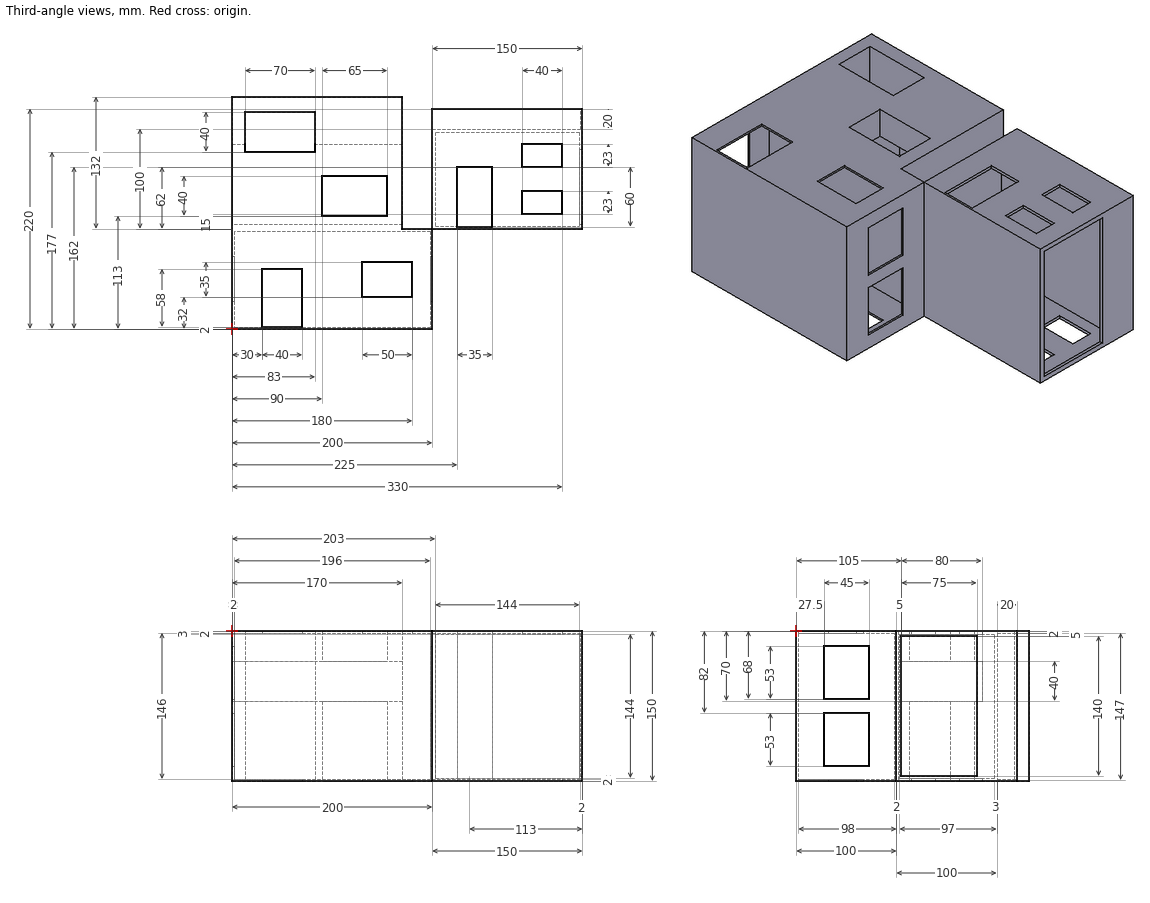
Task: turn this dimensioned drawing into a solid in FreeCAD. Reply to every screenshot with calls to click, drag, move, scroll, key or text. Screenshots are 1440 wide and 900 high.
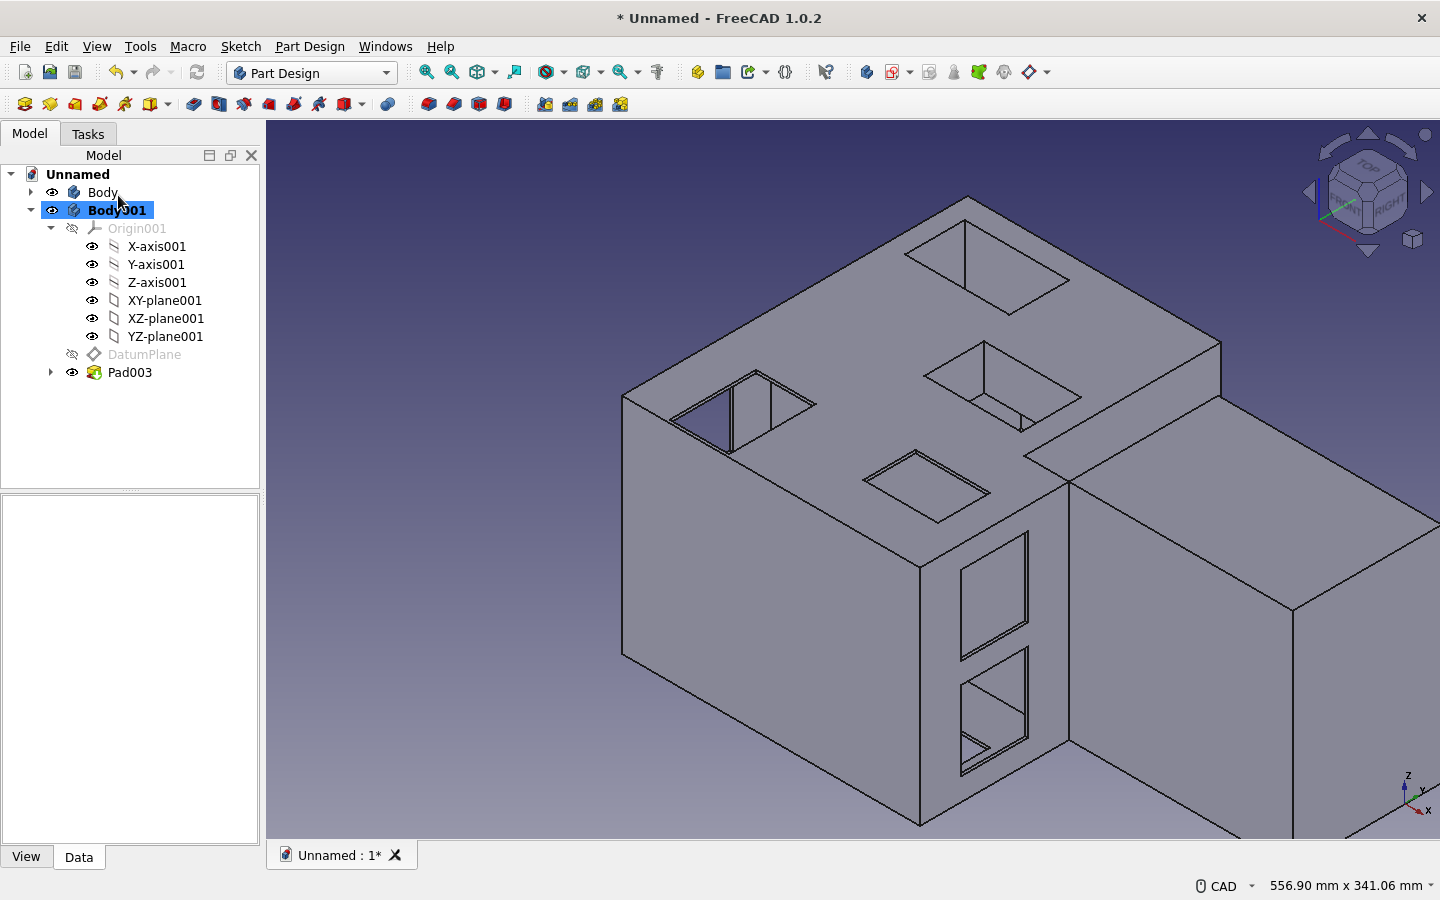
click(427, 72)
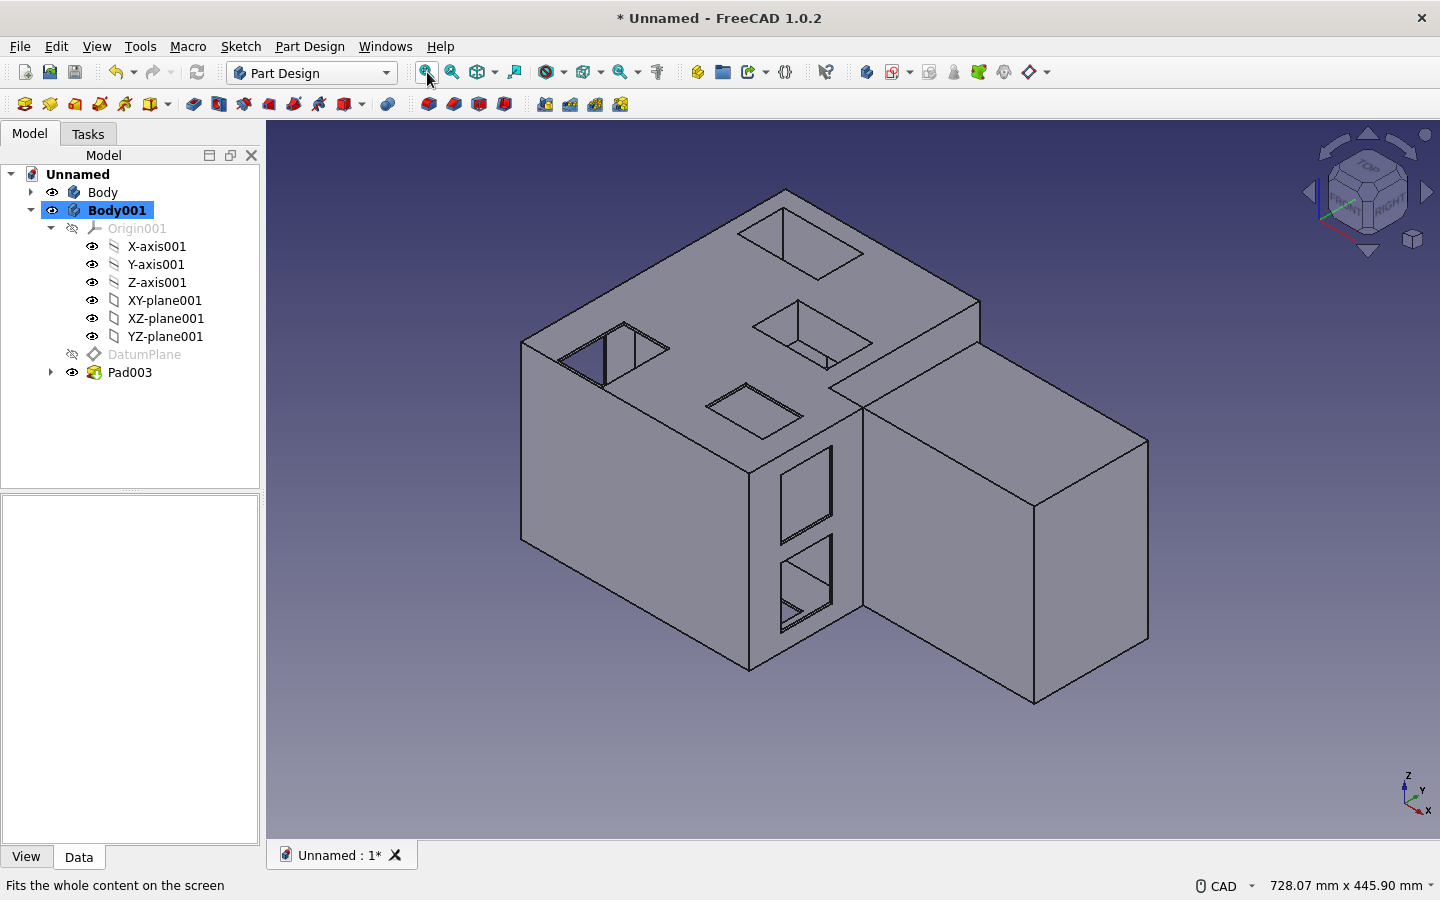
key(4)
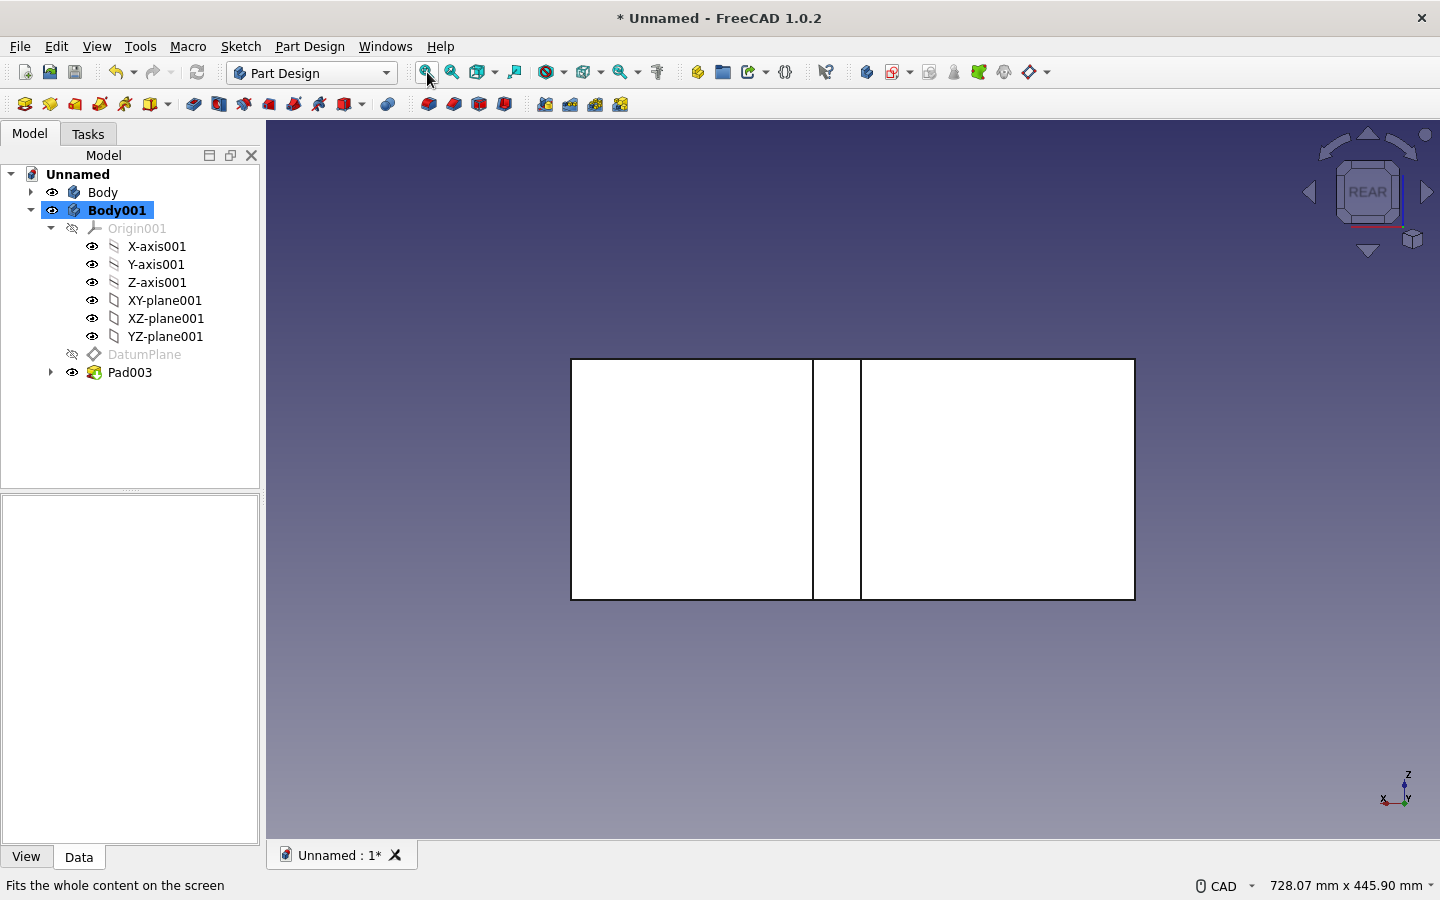
click(427, 72)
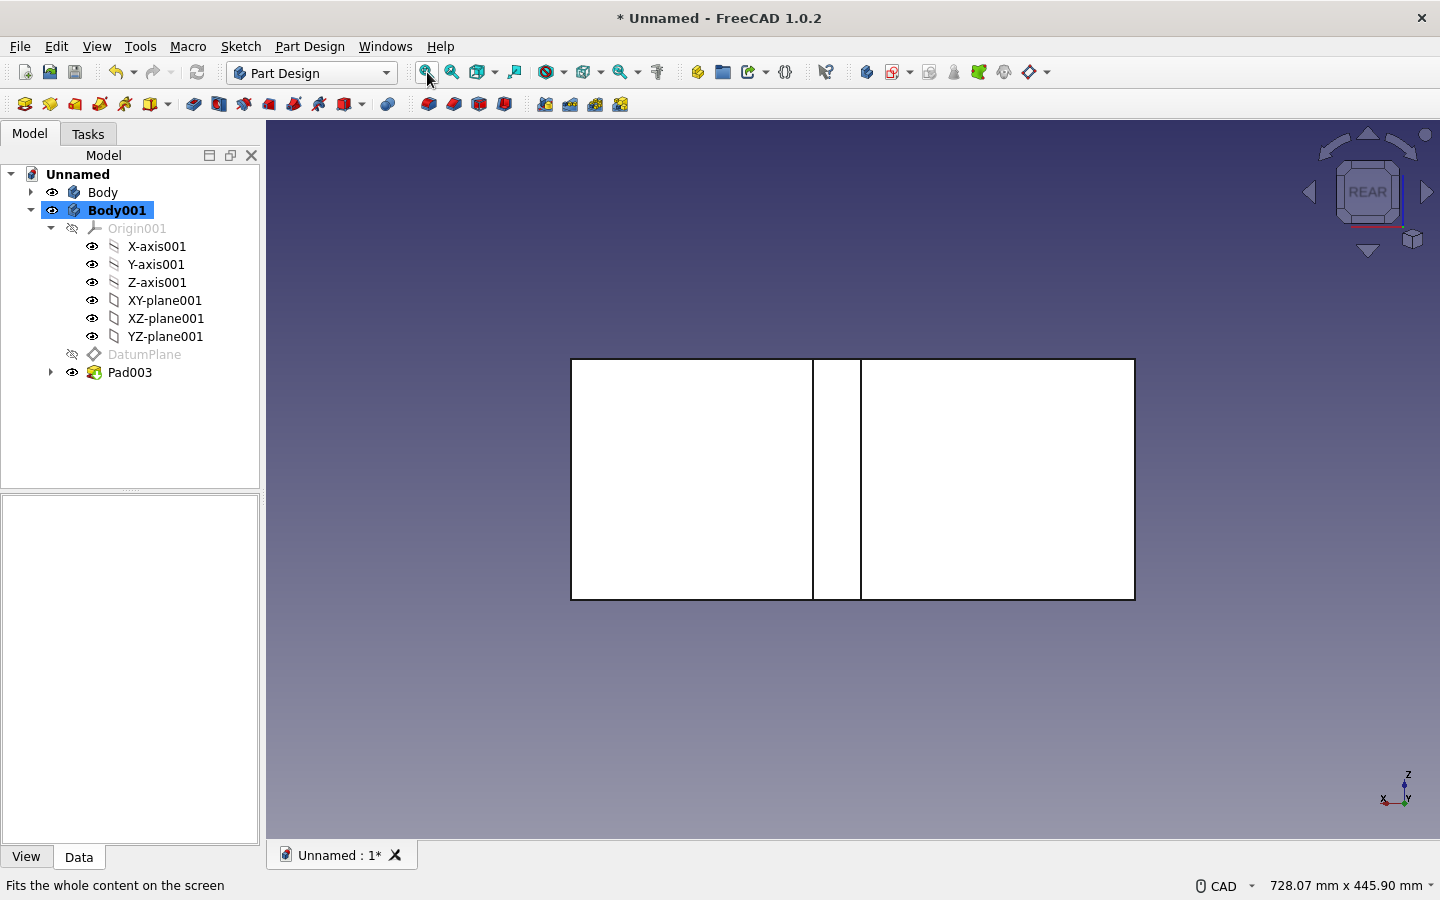
click(692, 479)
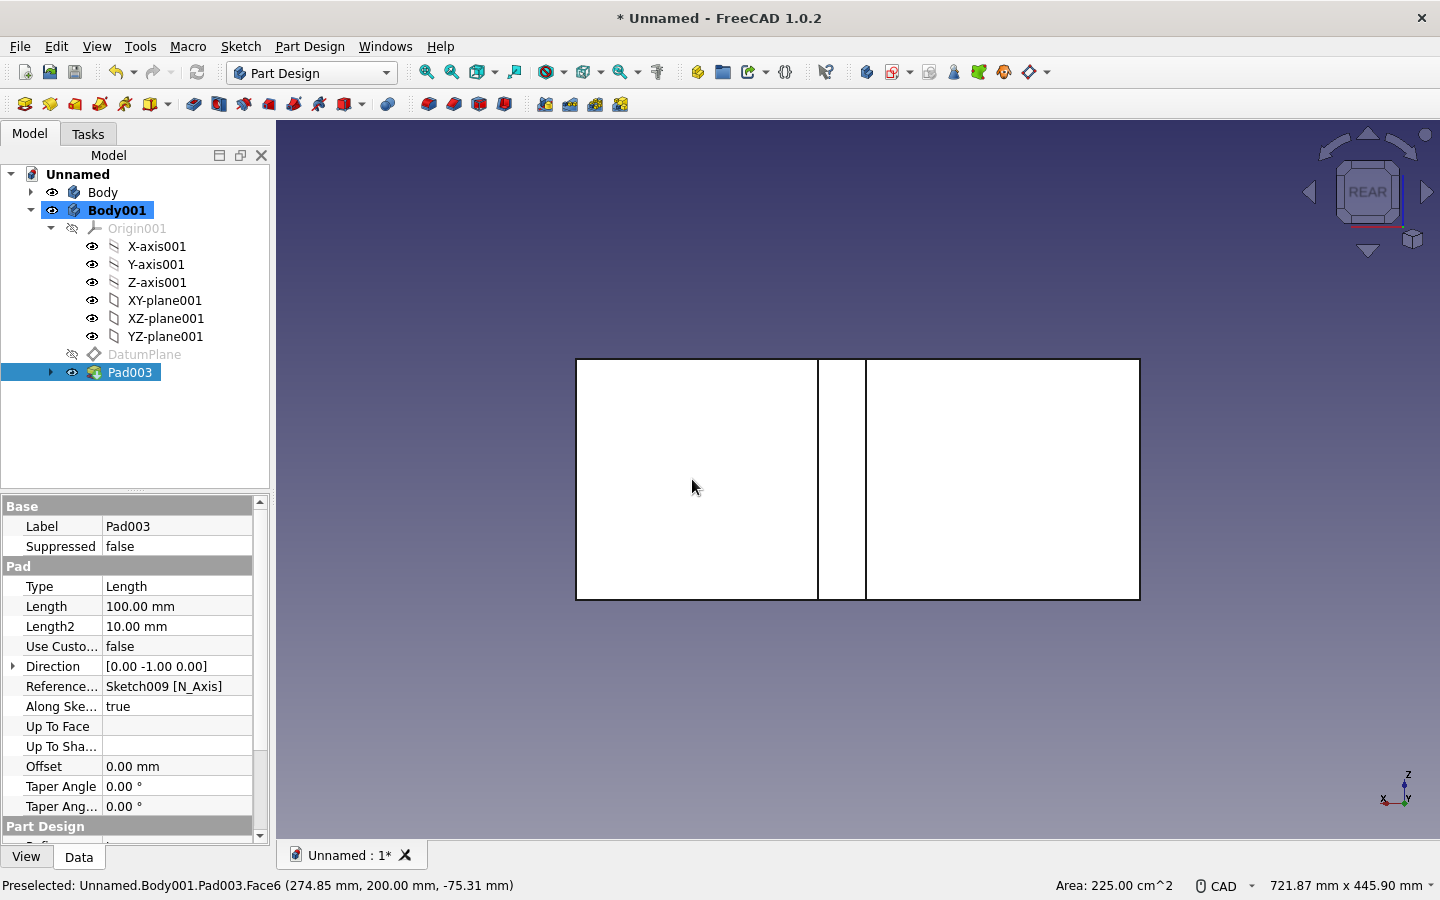
click(892, 72)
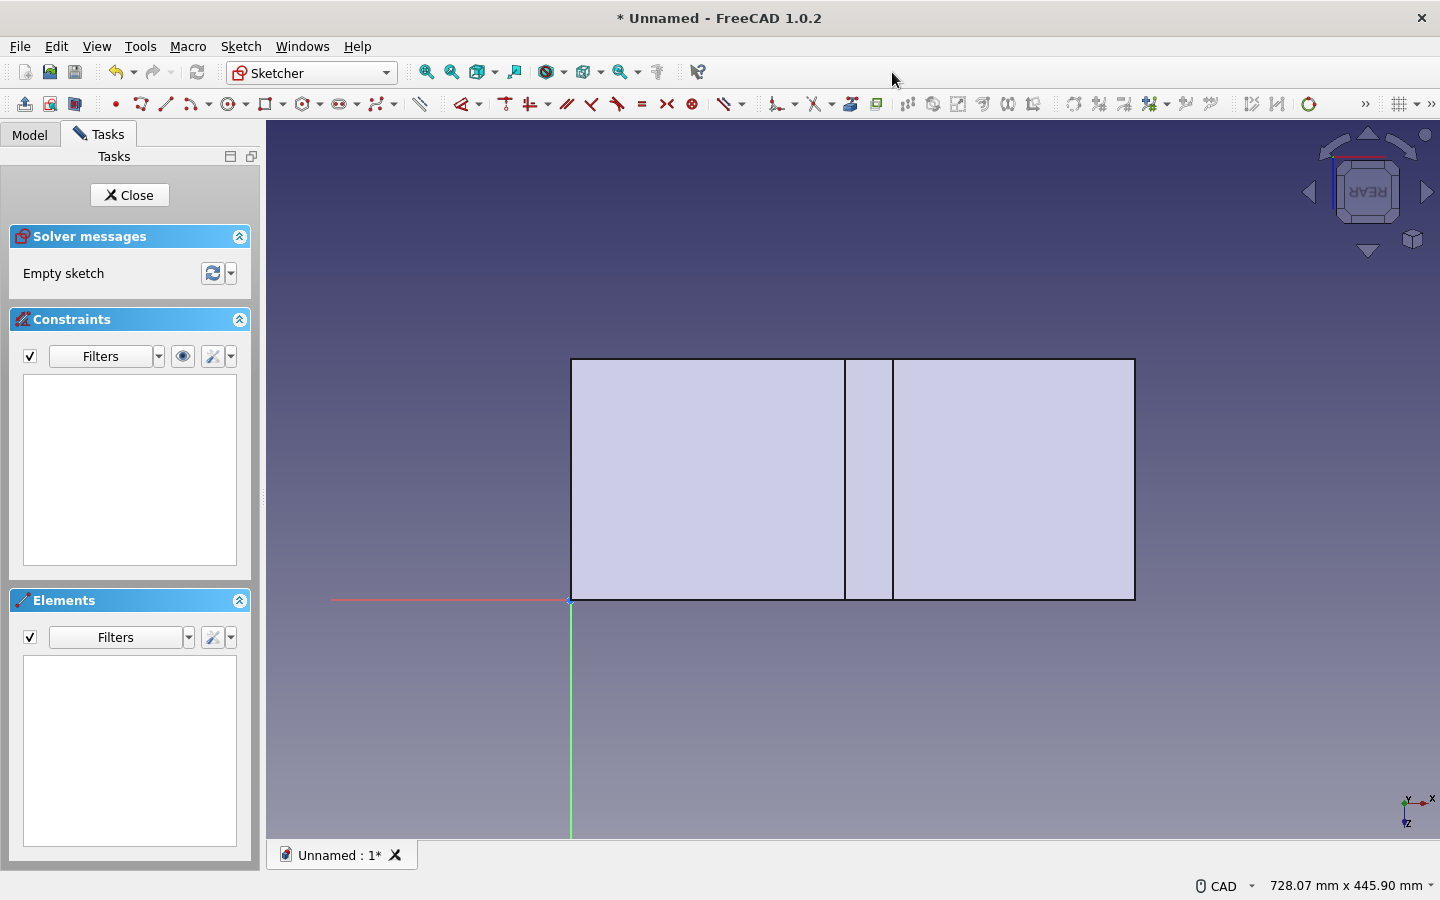
click(264, 104)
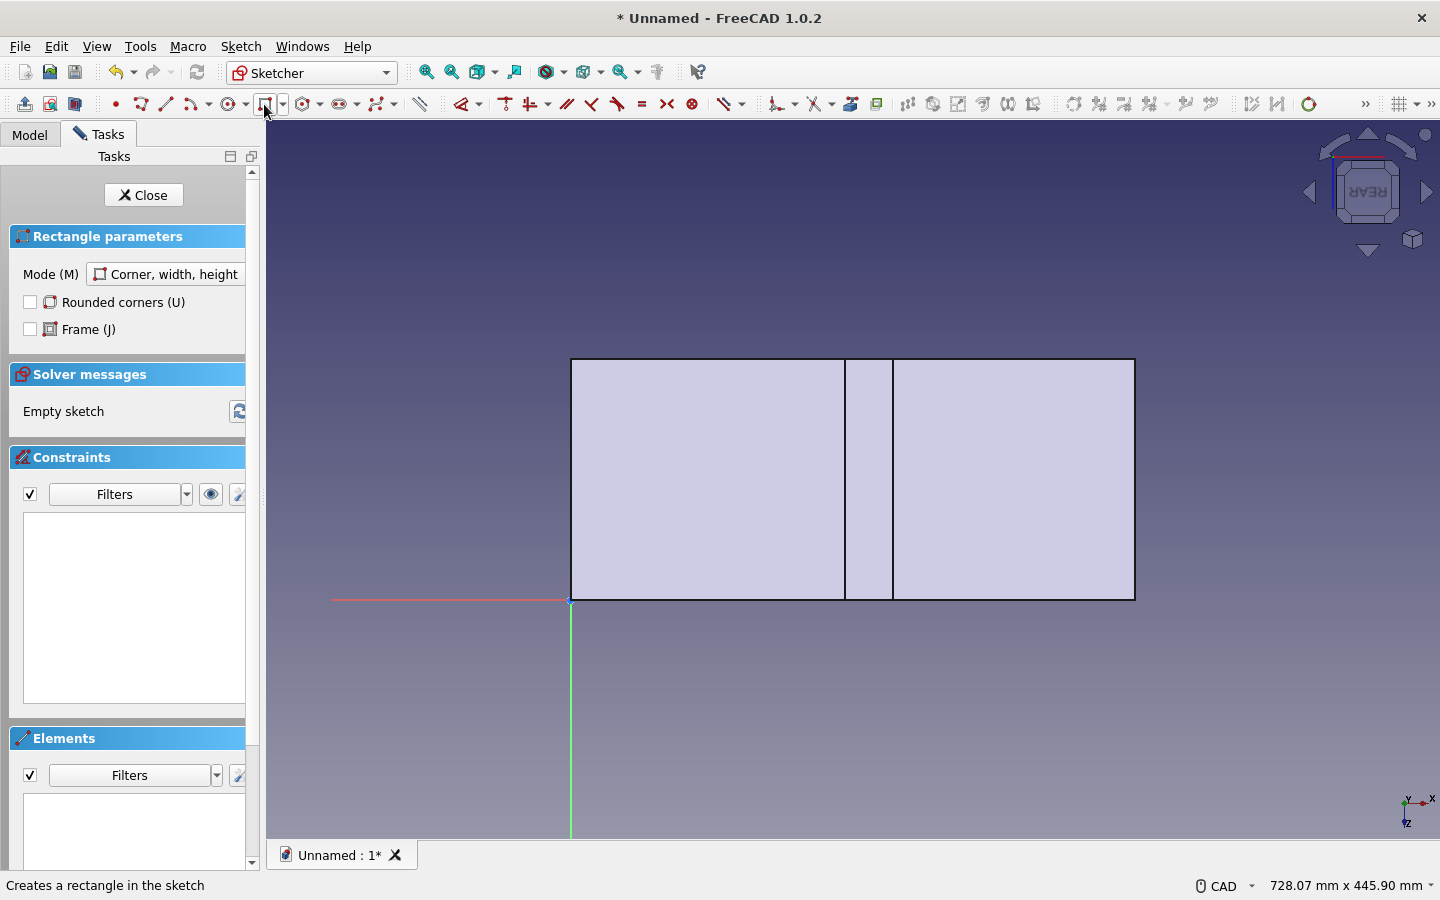
click(898, 363)